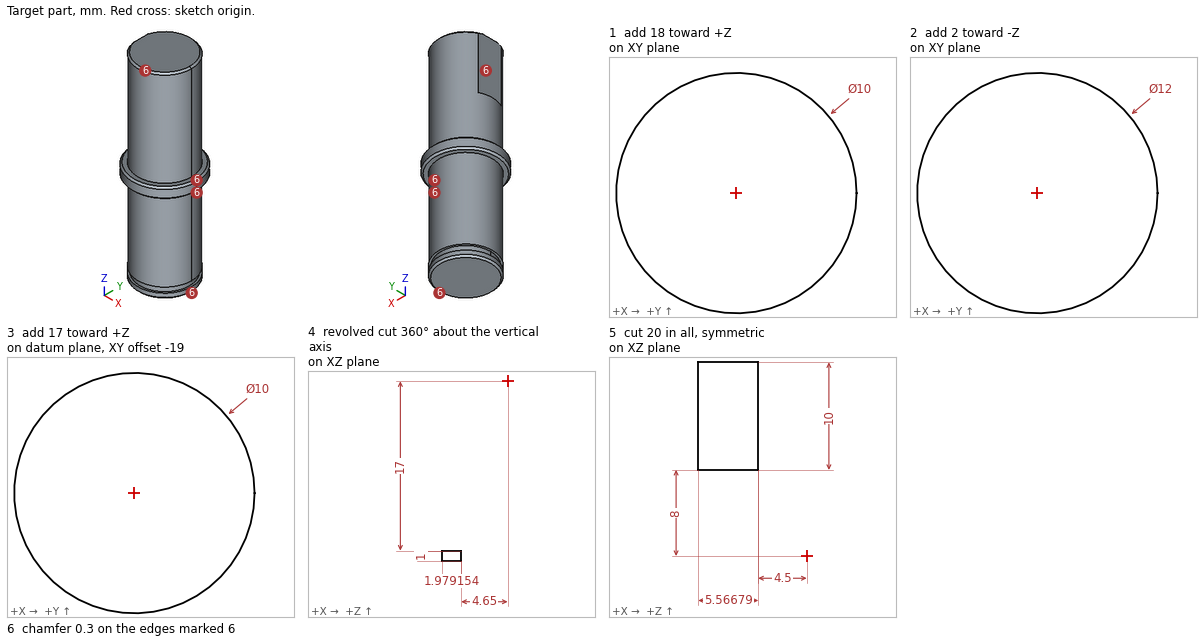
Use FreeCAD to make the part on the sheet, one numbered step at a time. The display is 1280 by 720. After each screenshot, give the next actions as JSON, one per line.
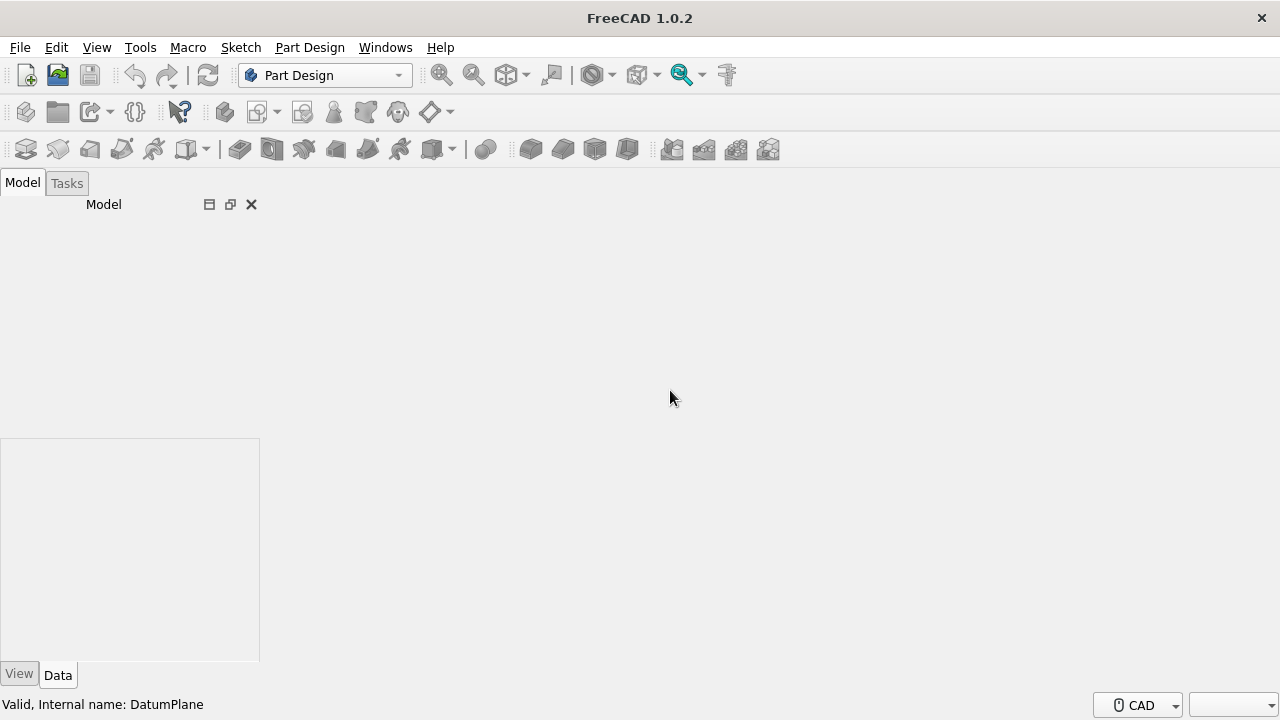
{"action": "left_click", "coordinate": [26, 76]}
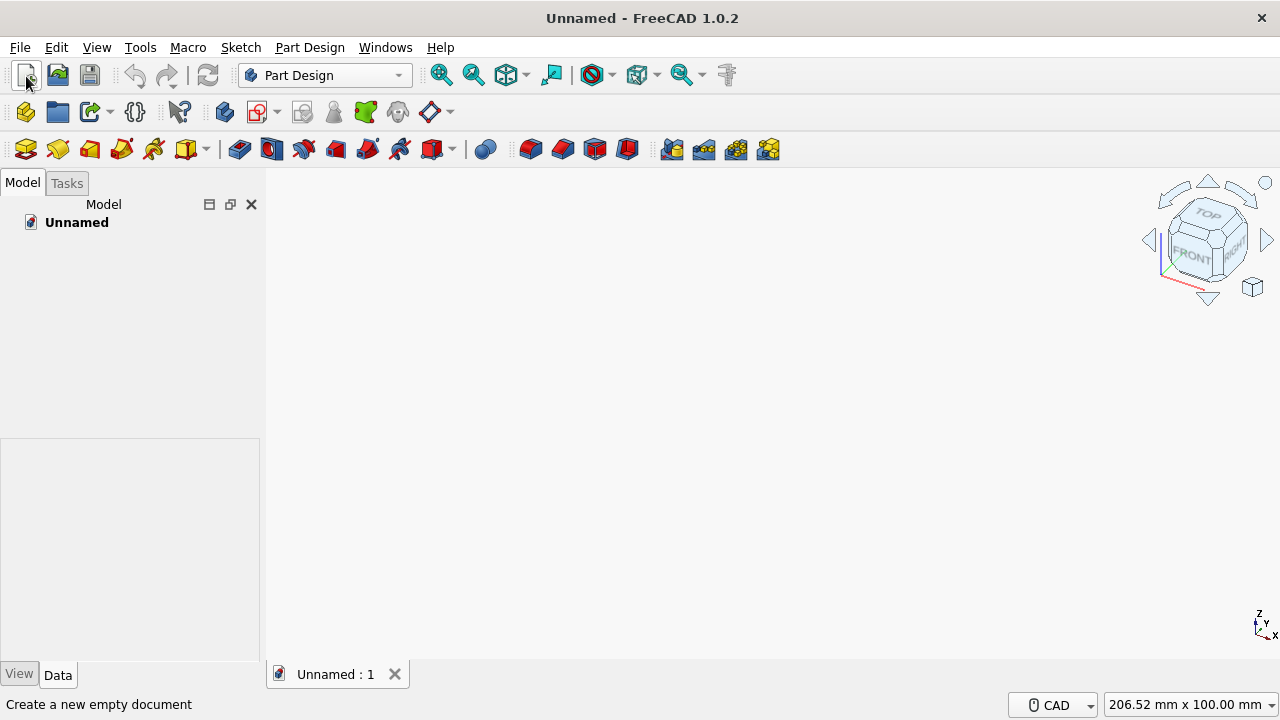
{"action": "left_click", "coordinate": [258, 112]}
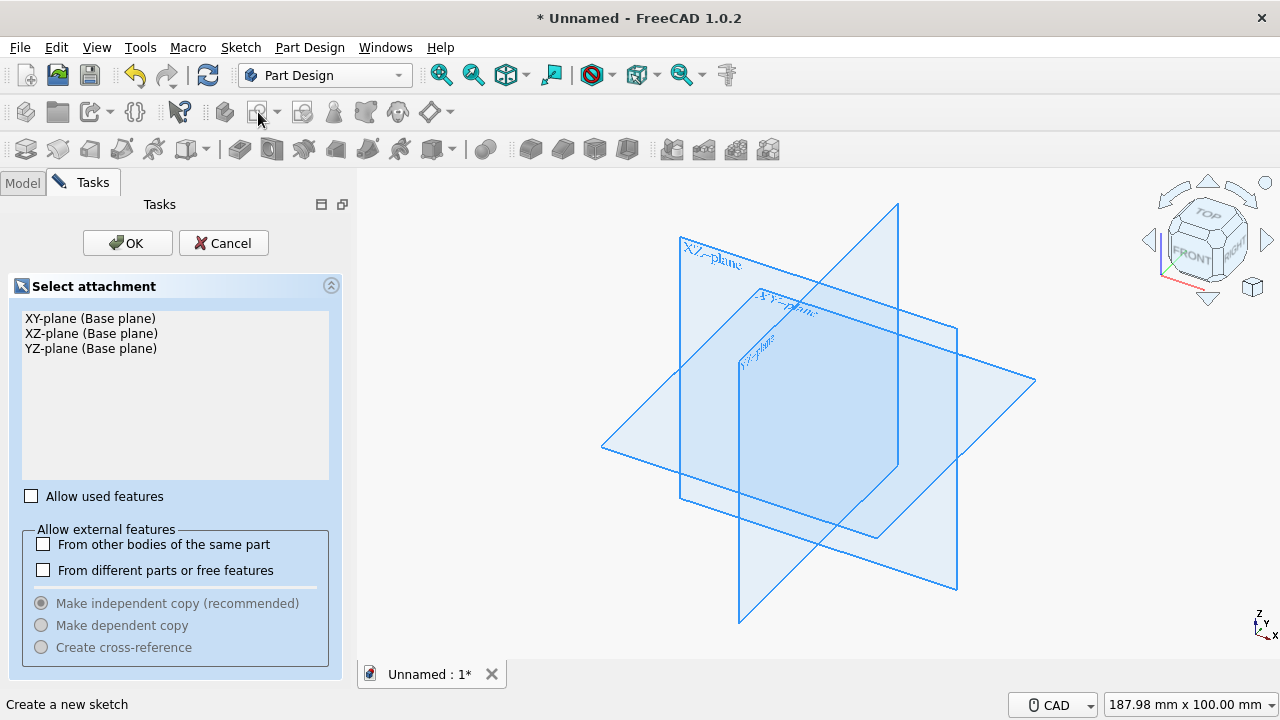
{"action": "left_click", "coordinate": [82, 318]}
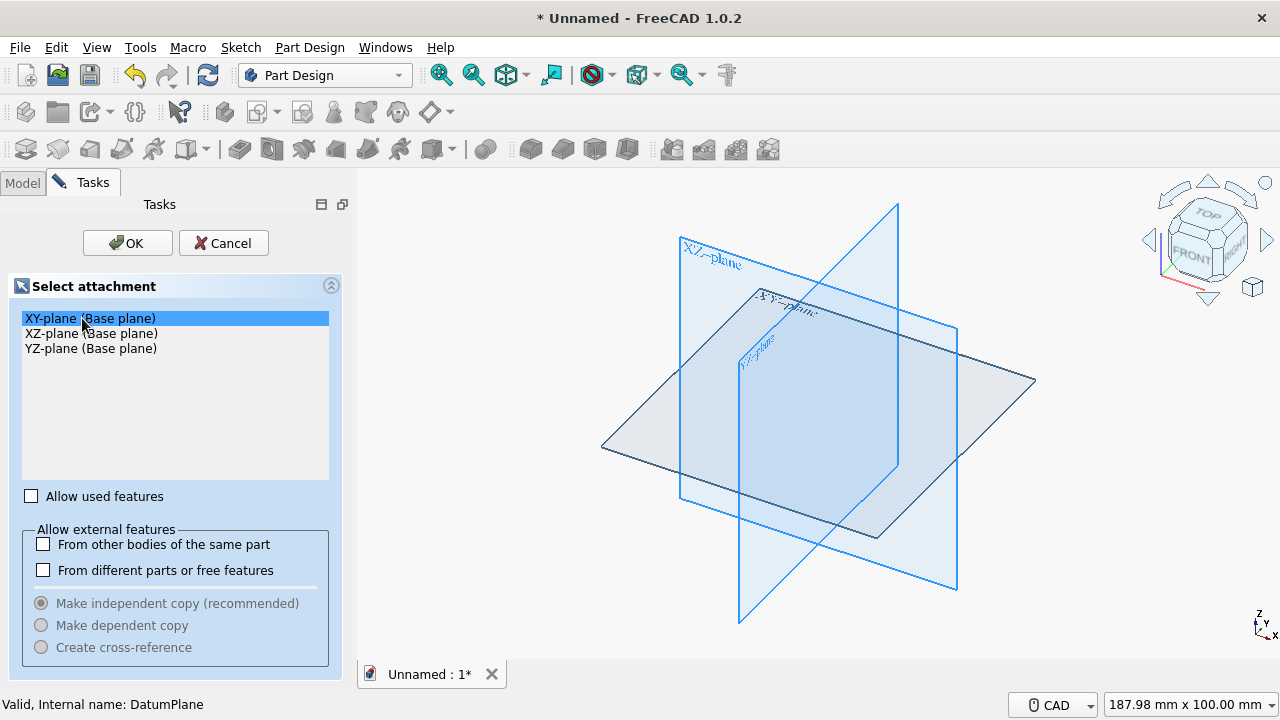
{"action": "left_click", "coordinate": [128, 243]}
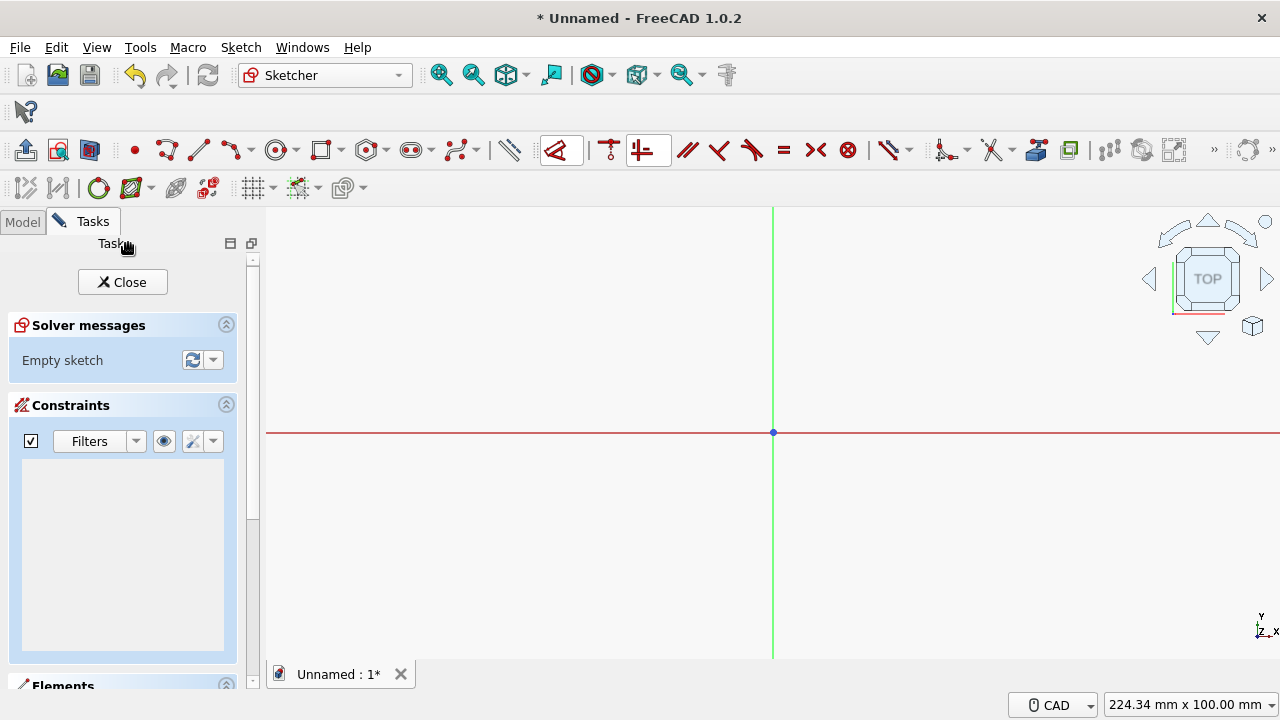
{"action": "scroll", "coordinate": [787, 433], "scroll_direction": "up", "scroll_amount": 9}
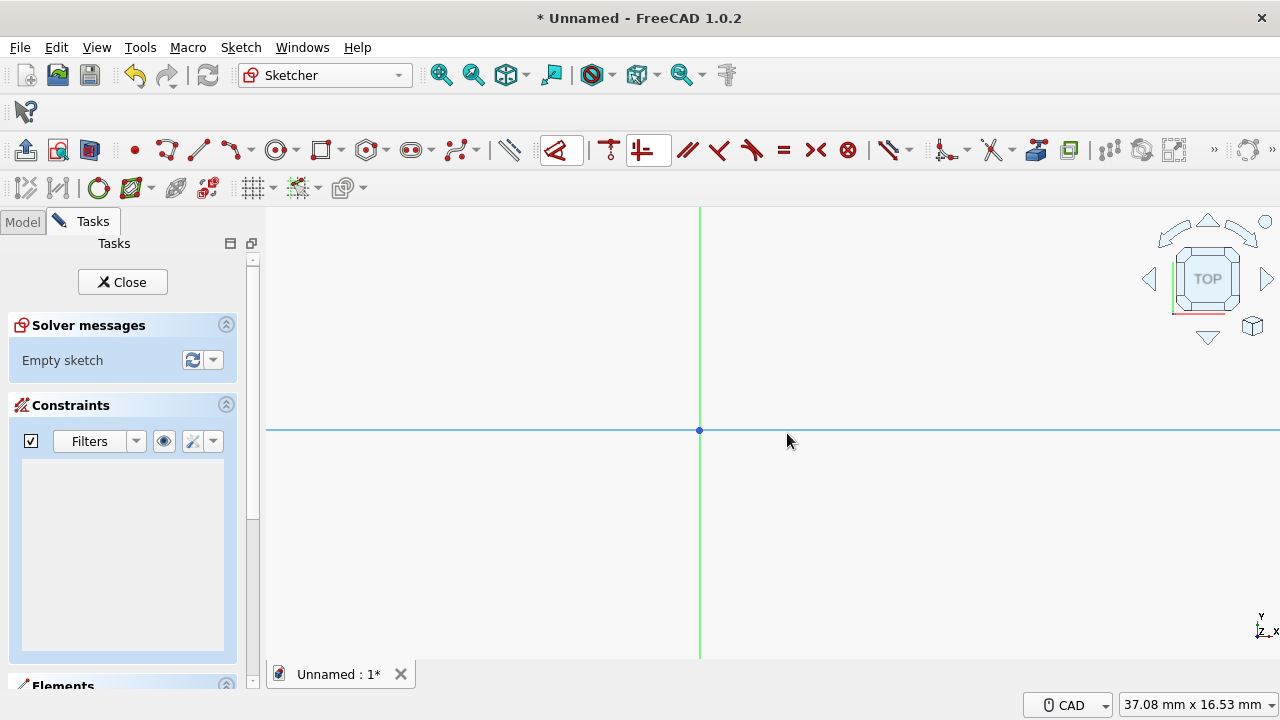
{"action": "left_click", "coordinate": [276, 150]}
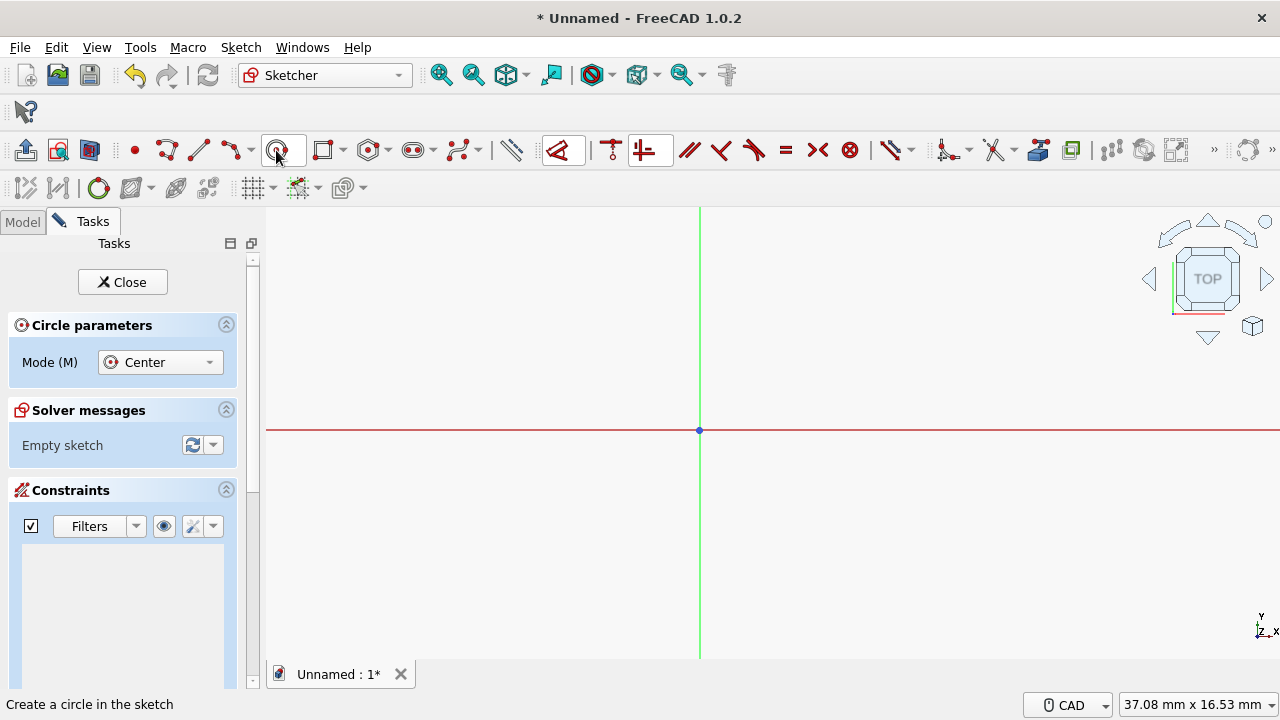
{"action": "left_click", "coordinate": [700, 430]}
{"action": "mouse_move", "coordinate": [796, 334]}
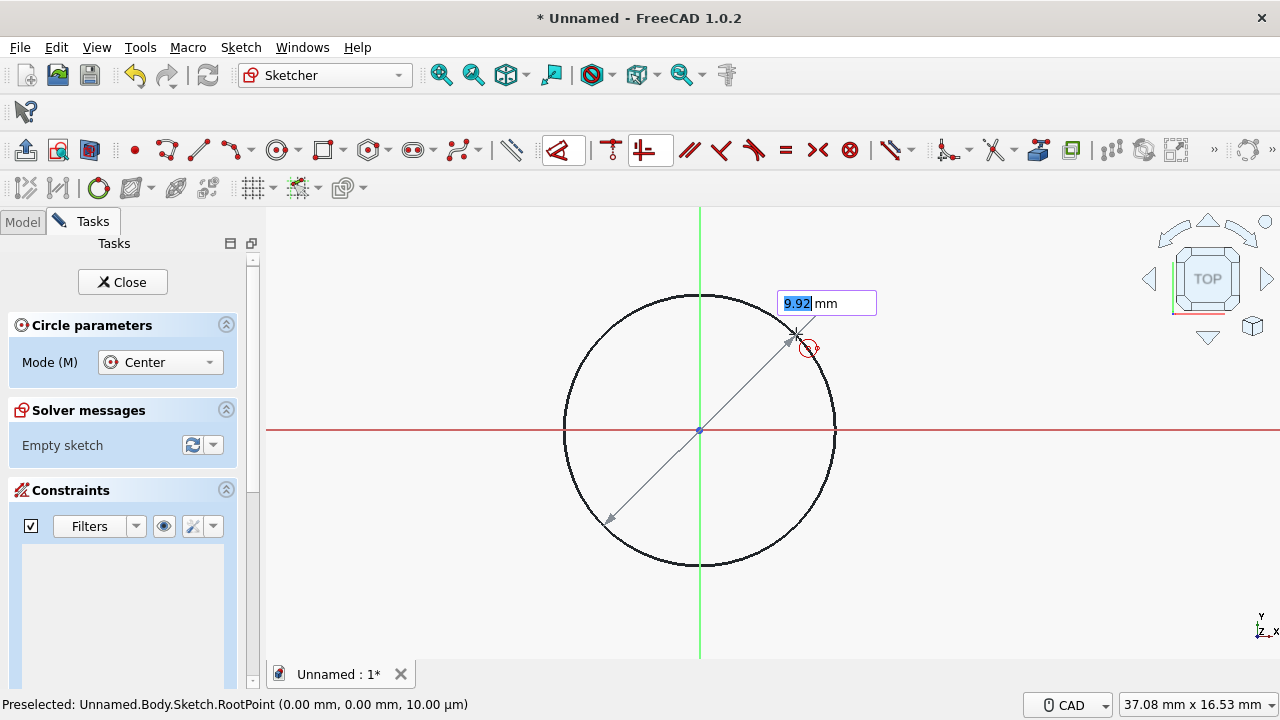
{"action": "type", "text": "10"}
{"action": "key", "text": "Return"}
{"action": "key", "text": "Escape"}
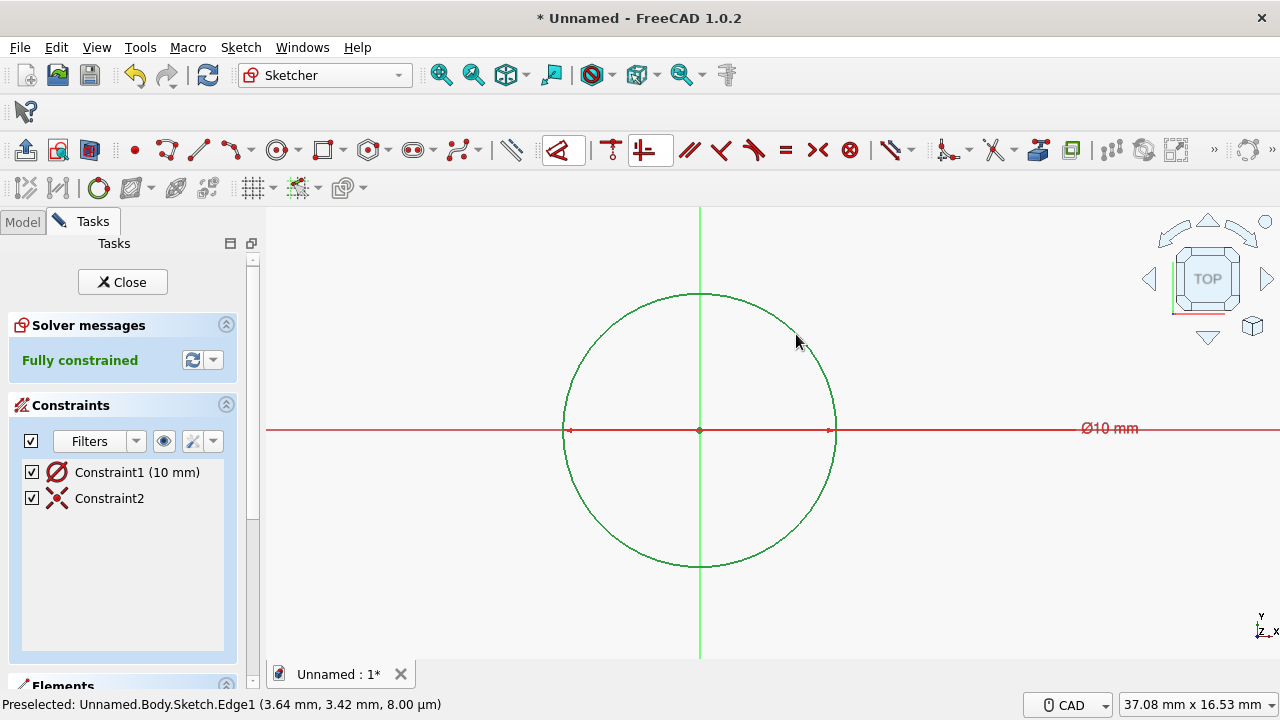
{"action": "left_click", "coordinate": [123, 282]}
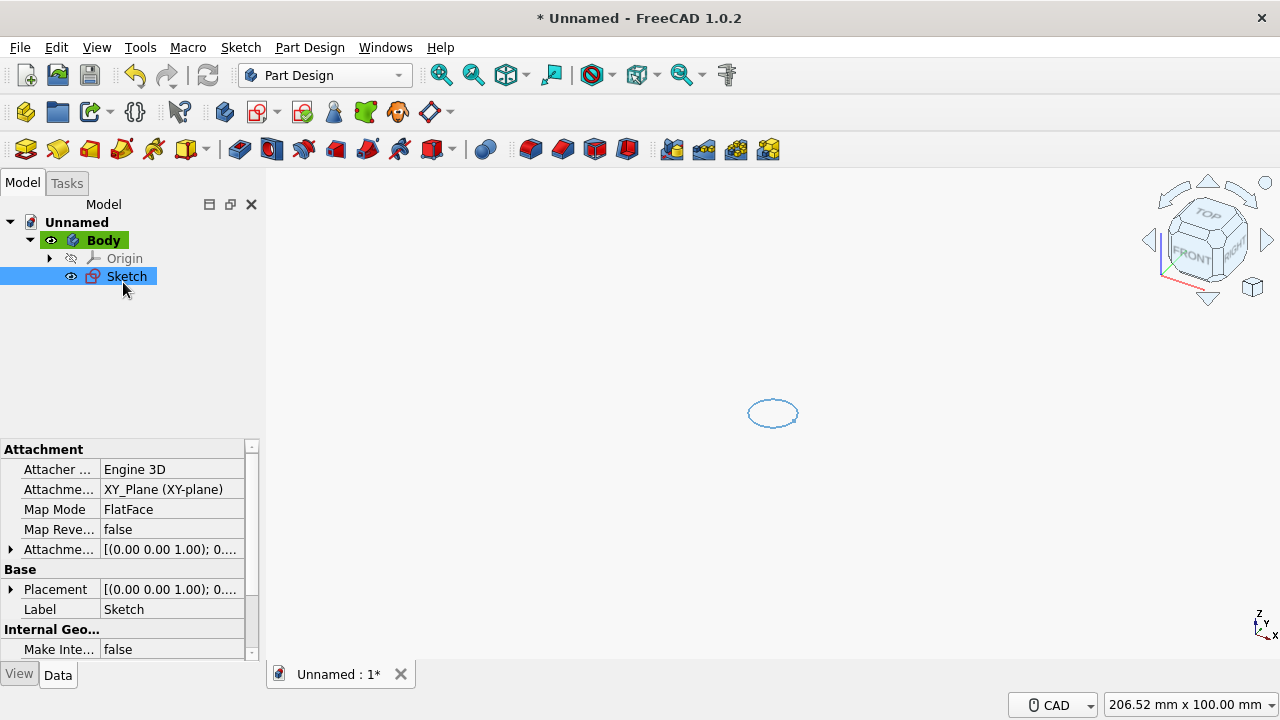
{"action": "left_click", "coordinate": [26, 150]}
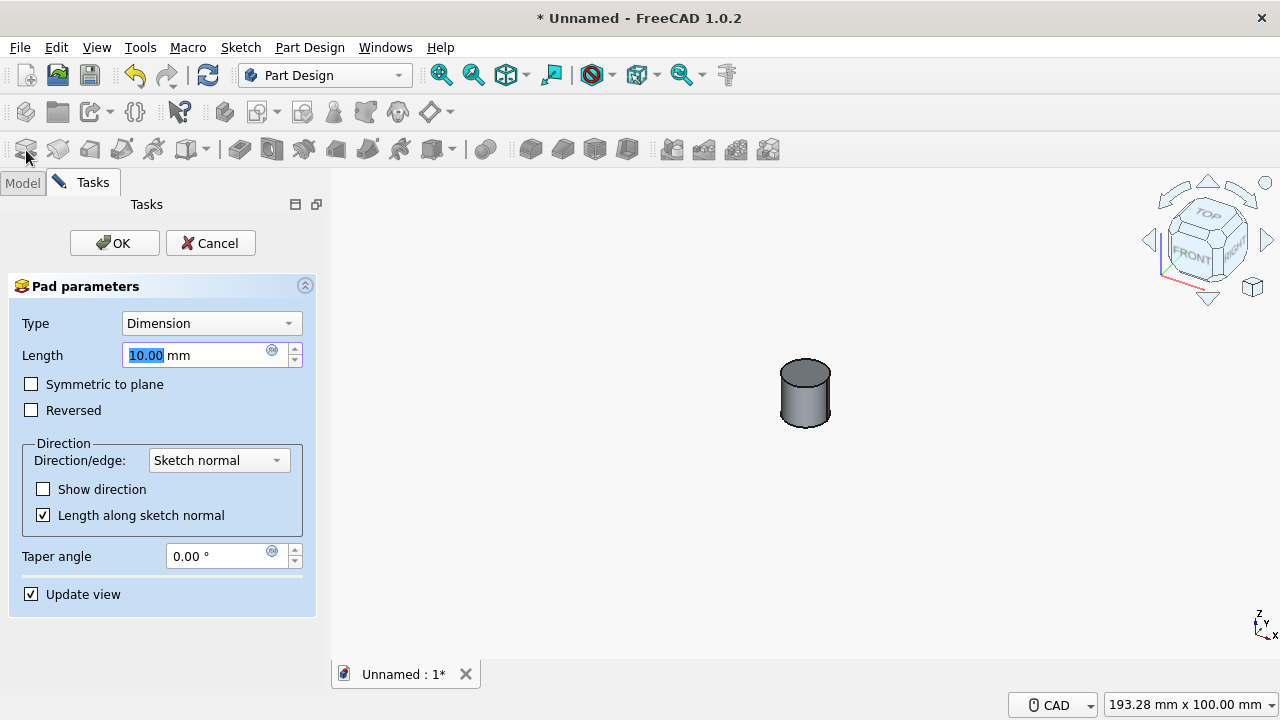
{"action": "type", "text": "18"}
{"action": "key", "text": "Tab"}